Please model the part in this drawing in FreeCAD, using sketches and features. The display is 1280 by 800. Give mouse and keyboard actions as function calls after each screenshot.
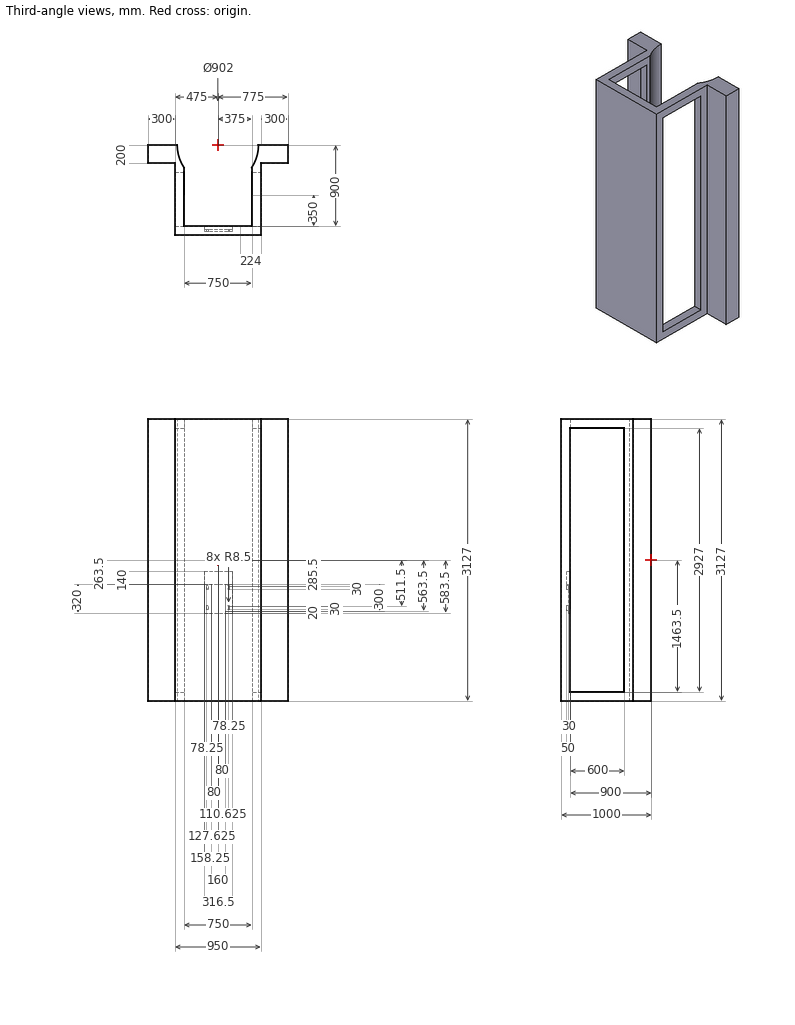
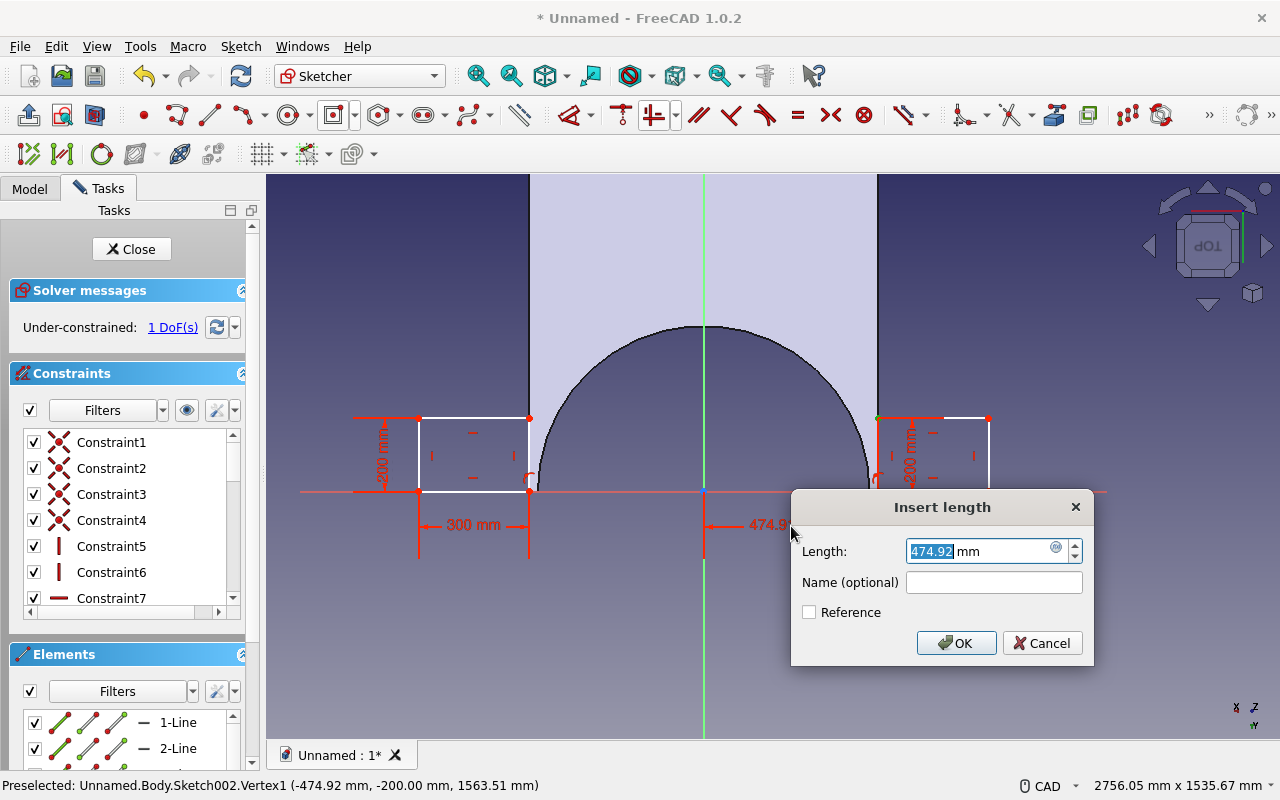
text(475)
key(Return)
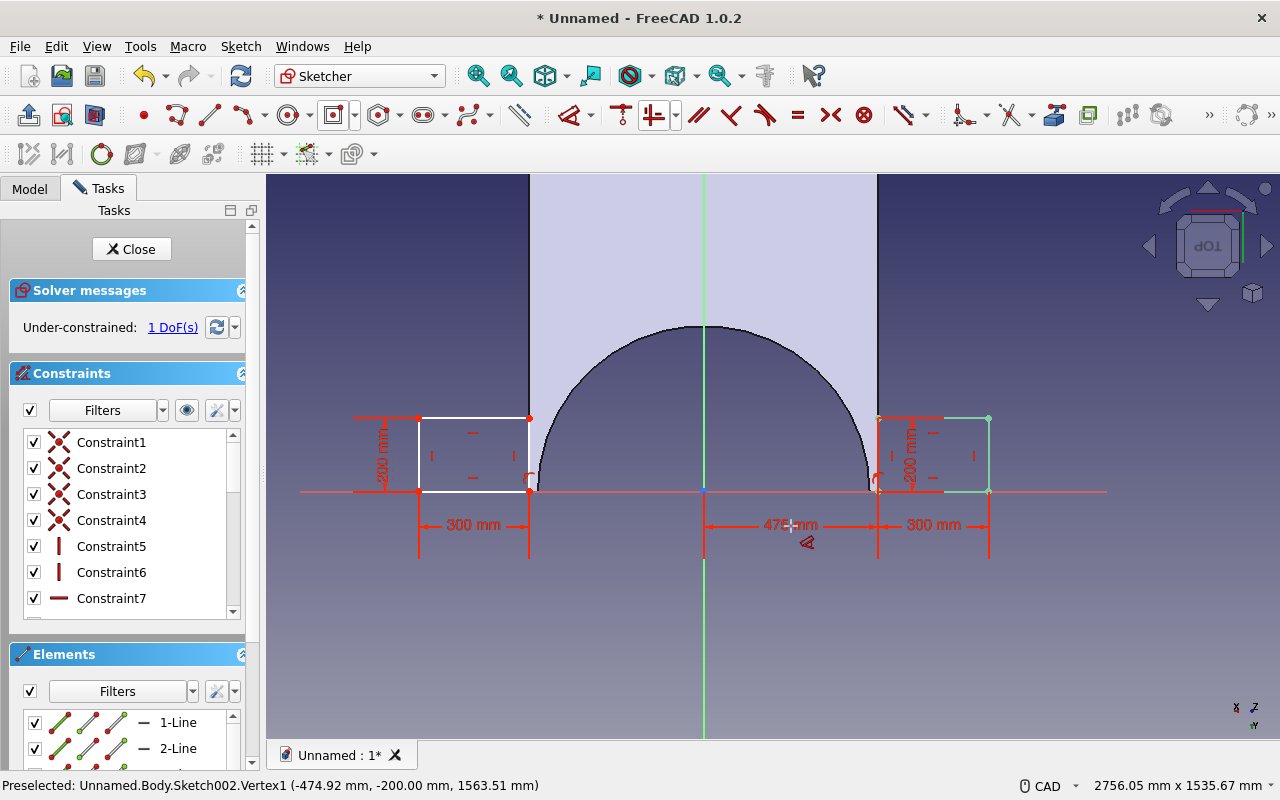
click(419, 418)
click(561, 526)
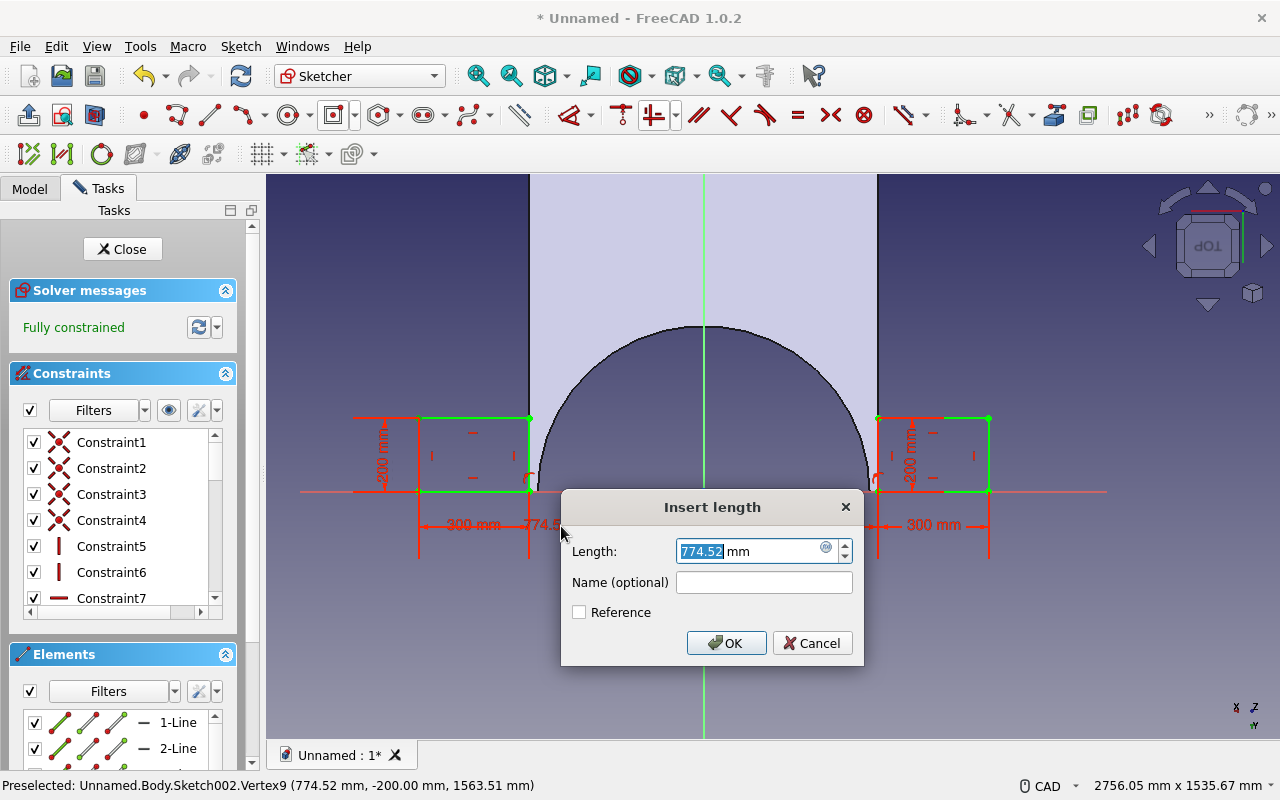
text(775)
key(Return)
key(Escape)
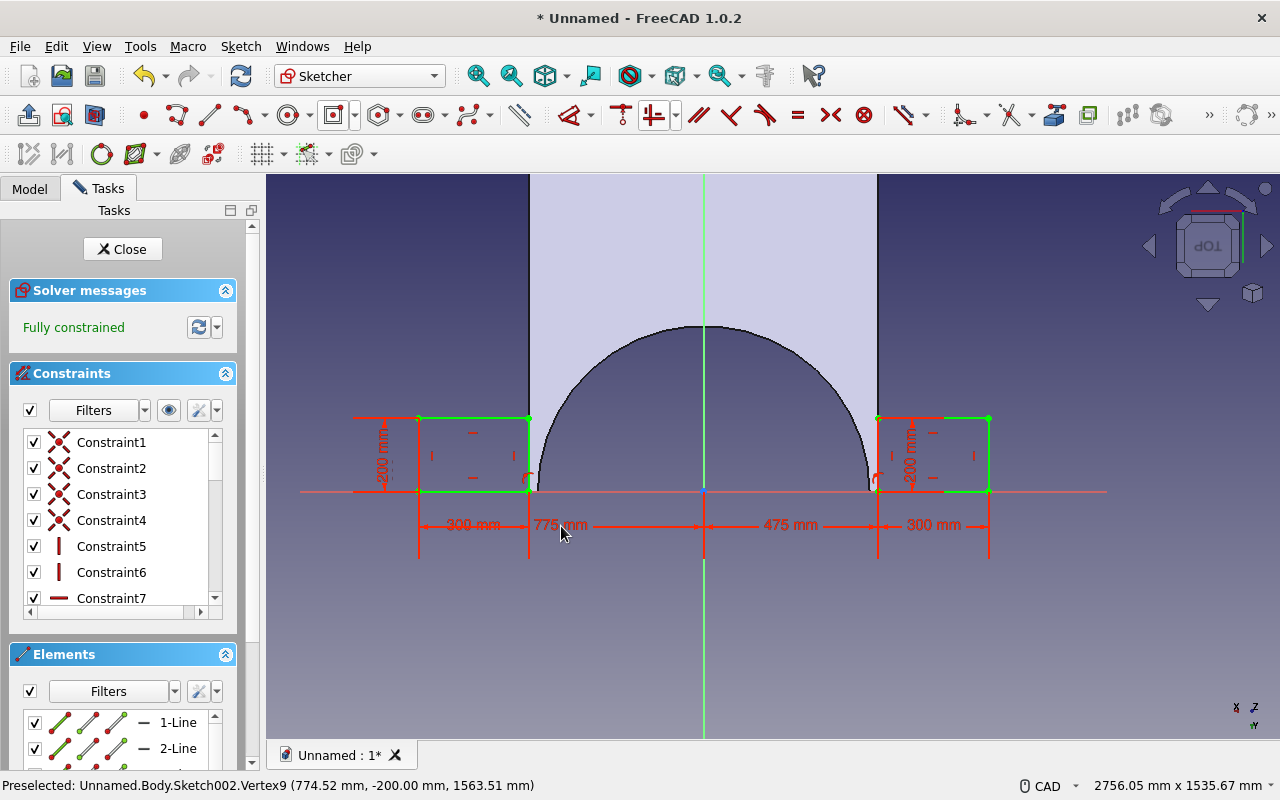
click(123, 249)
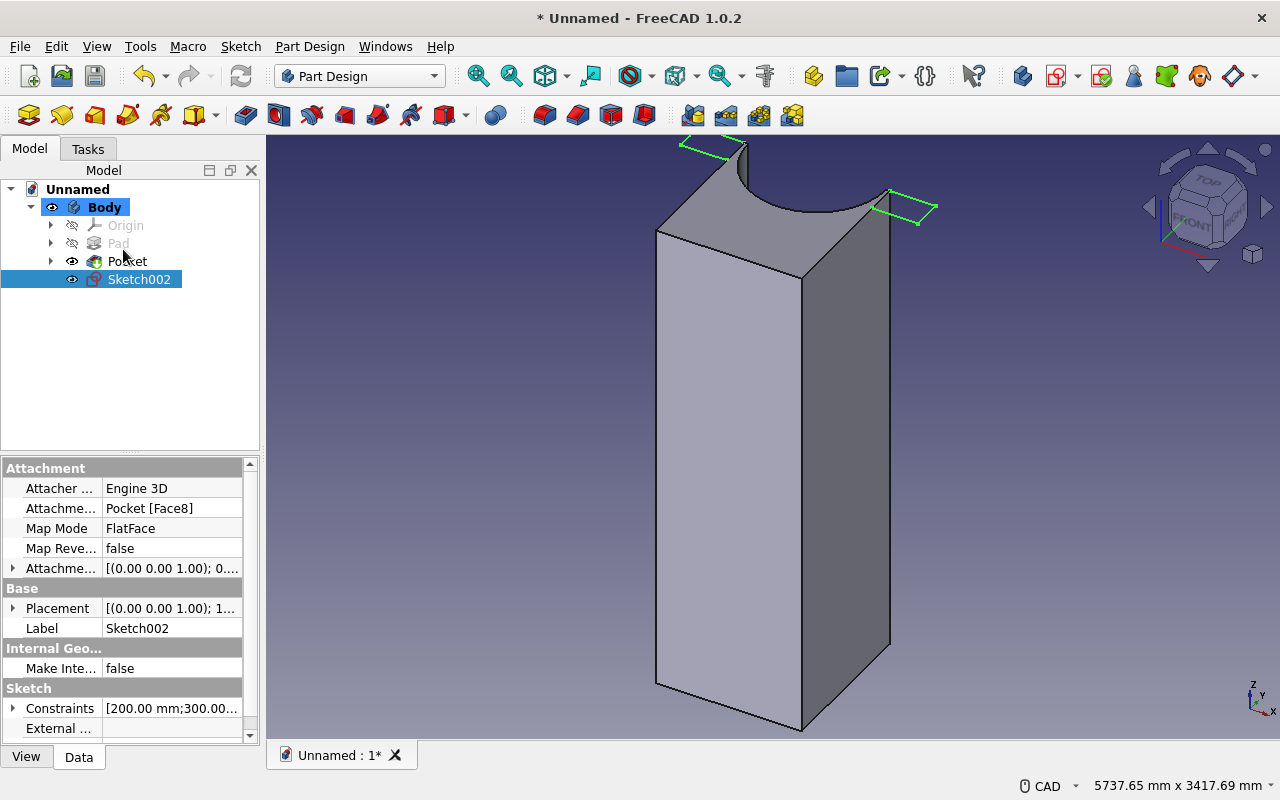
click(29, 116)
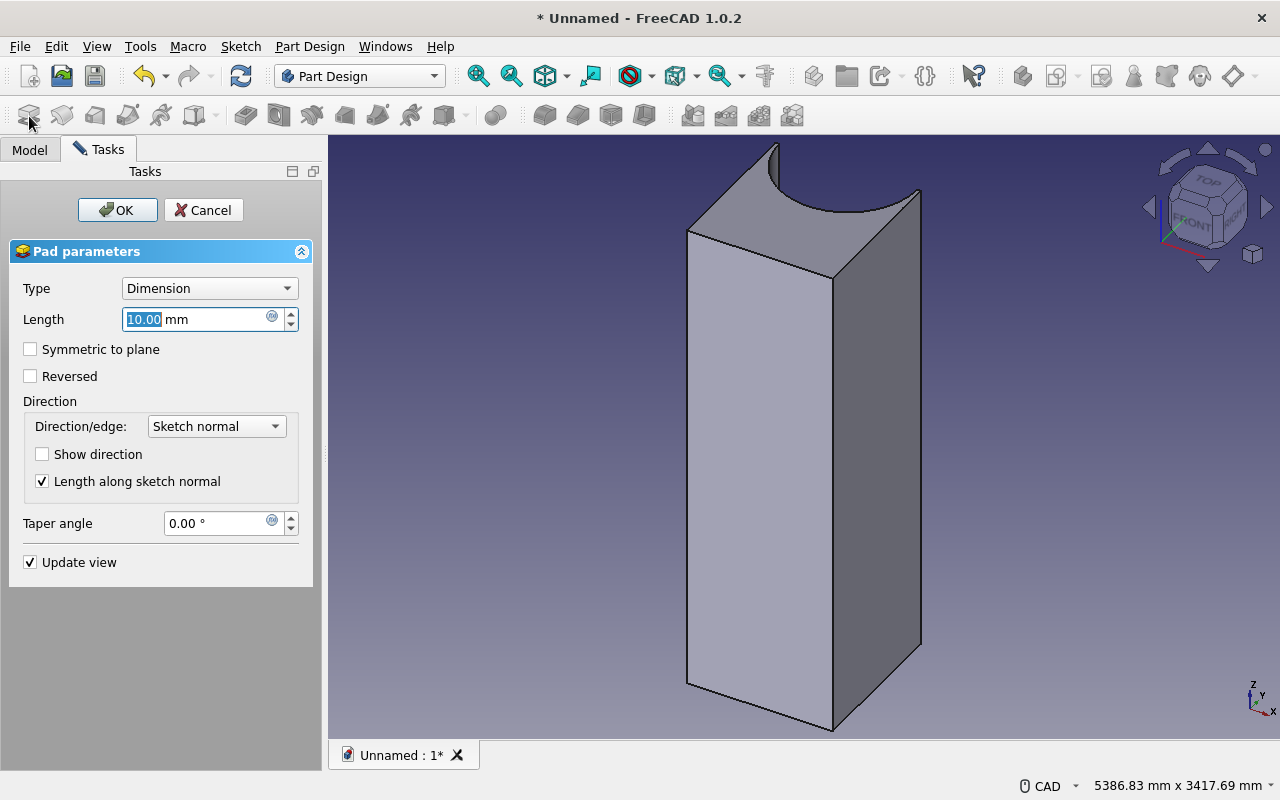
text(3127)
key(Tab)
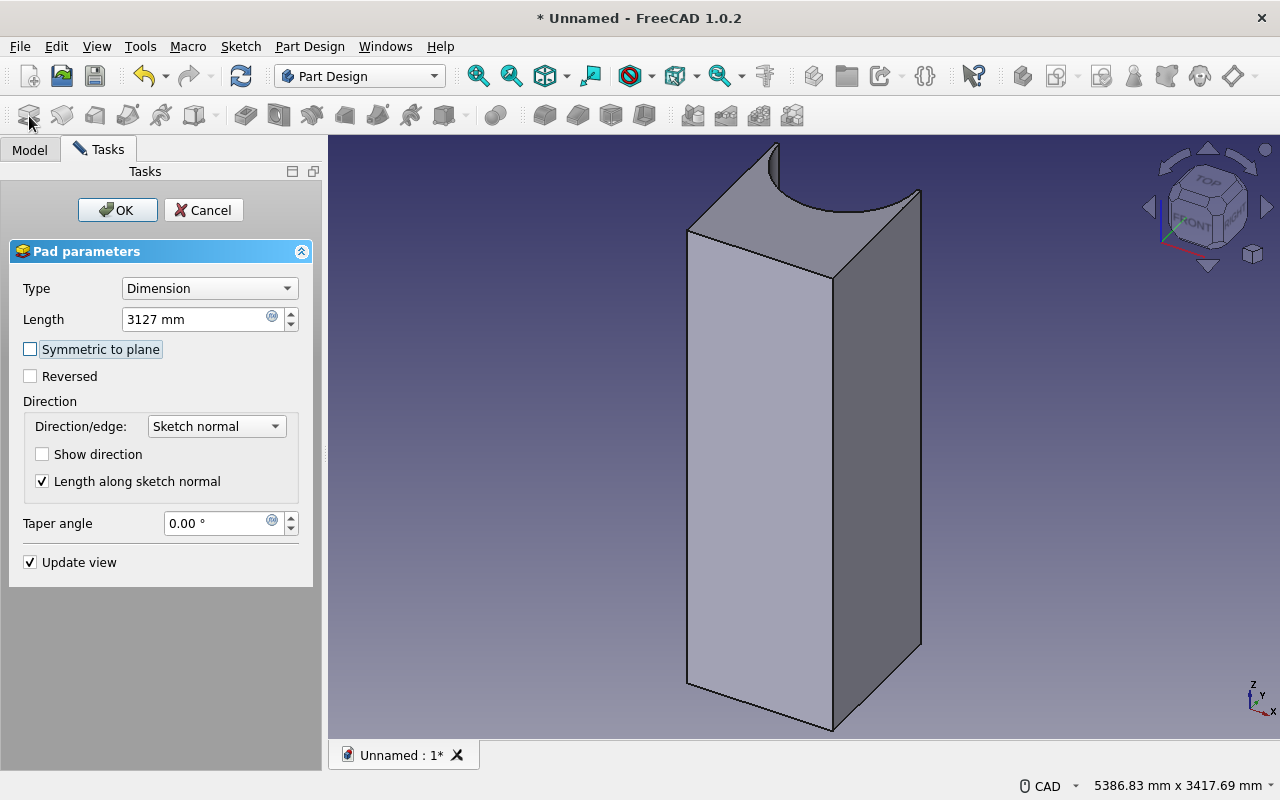
click(31, 376)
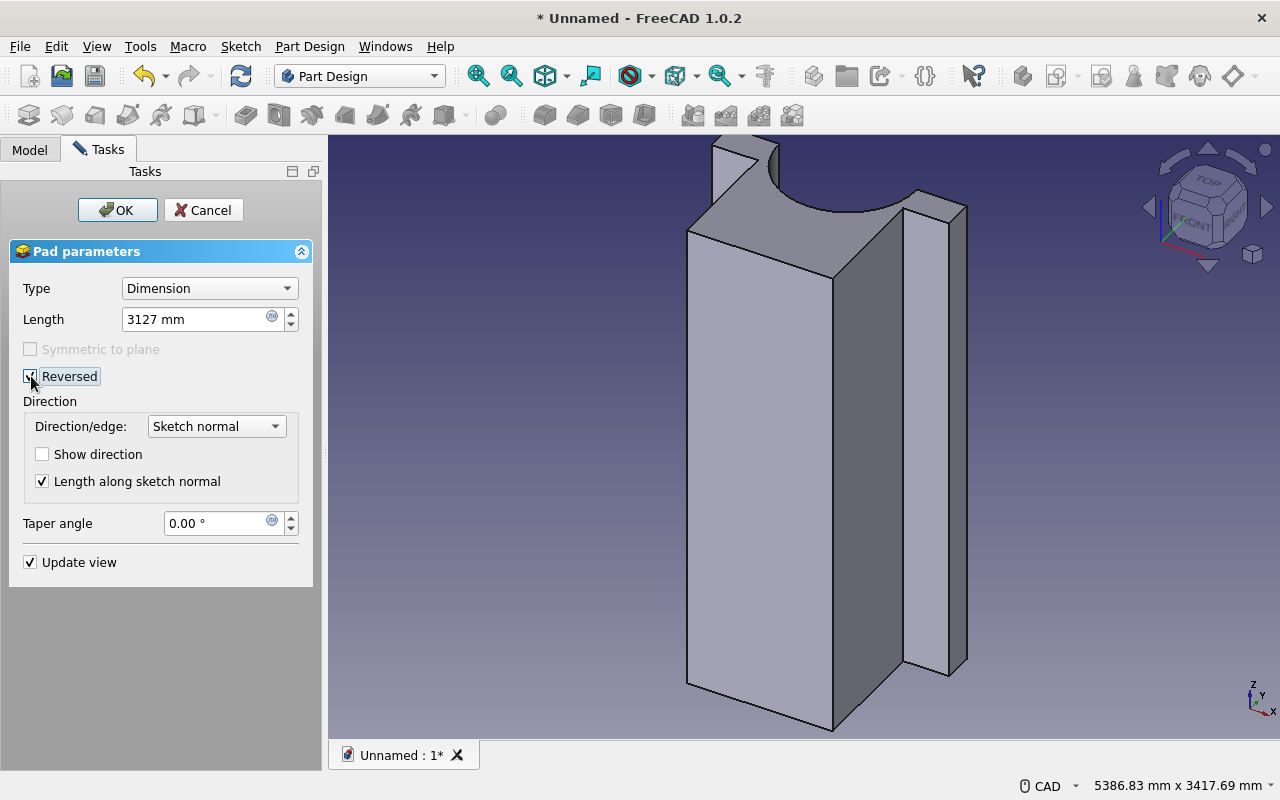
click(118, 210)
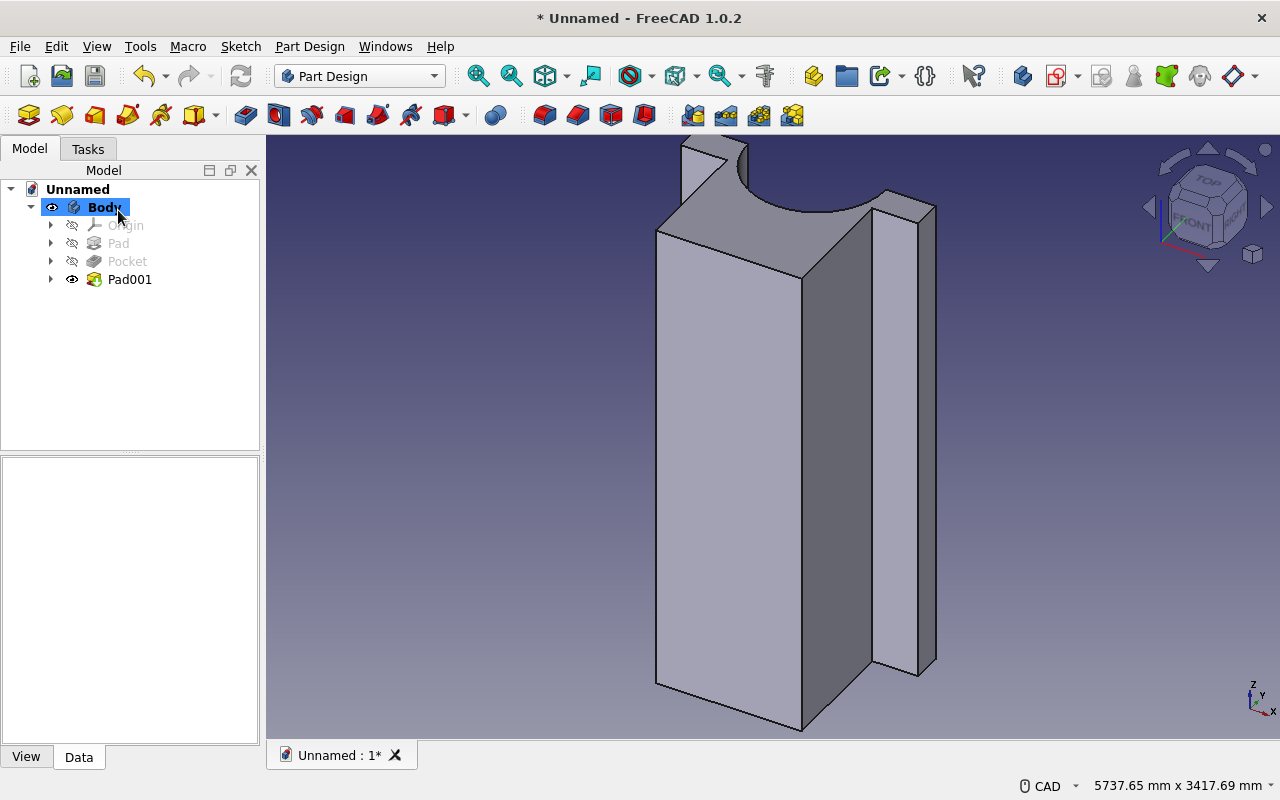
click(479, 76)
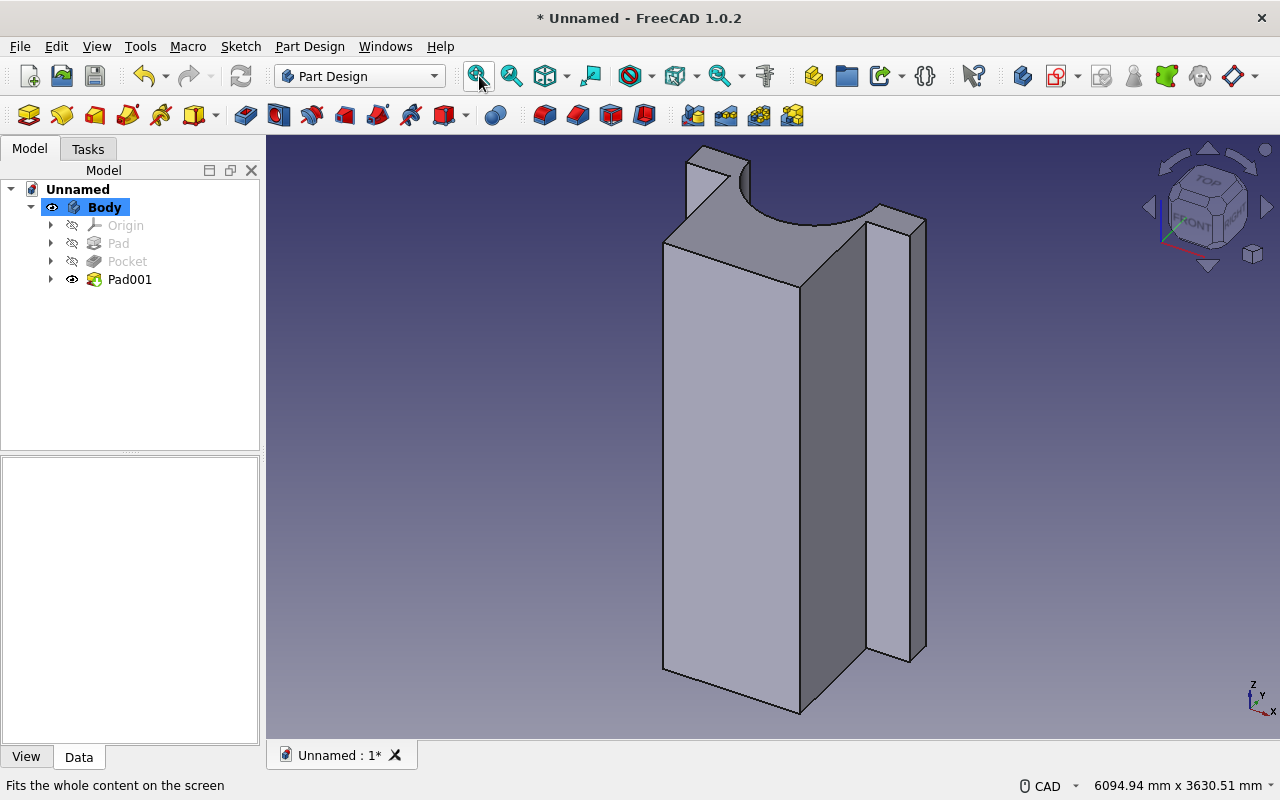
click(729, 224)